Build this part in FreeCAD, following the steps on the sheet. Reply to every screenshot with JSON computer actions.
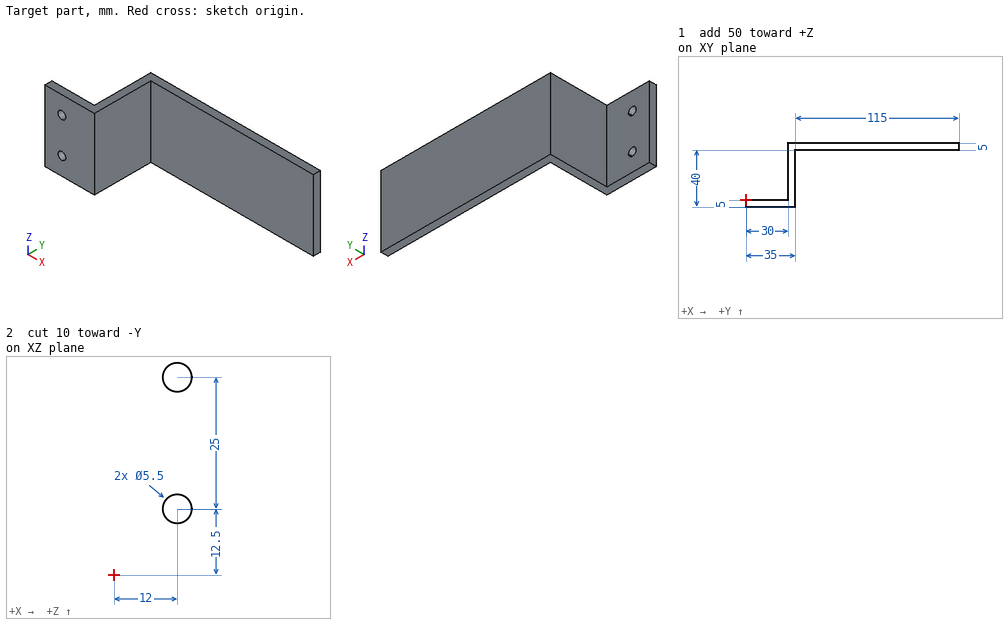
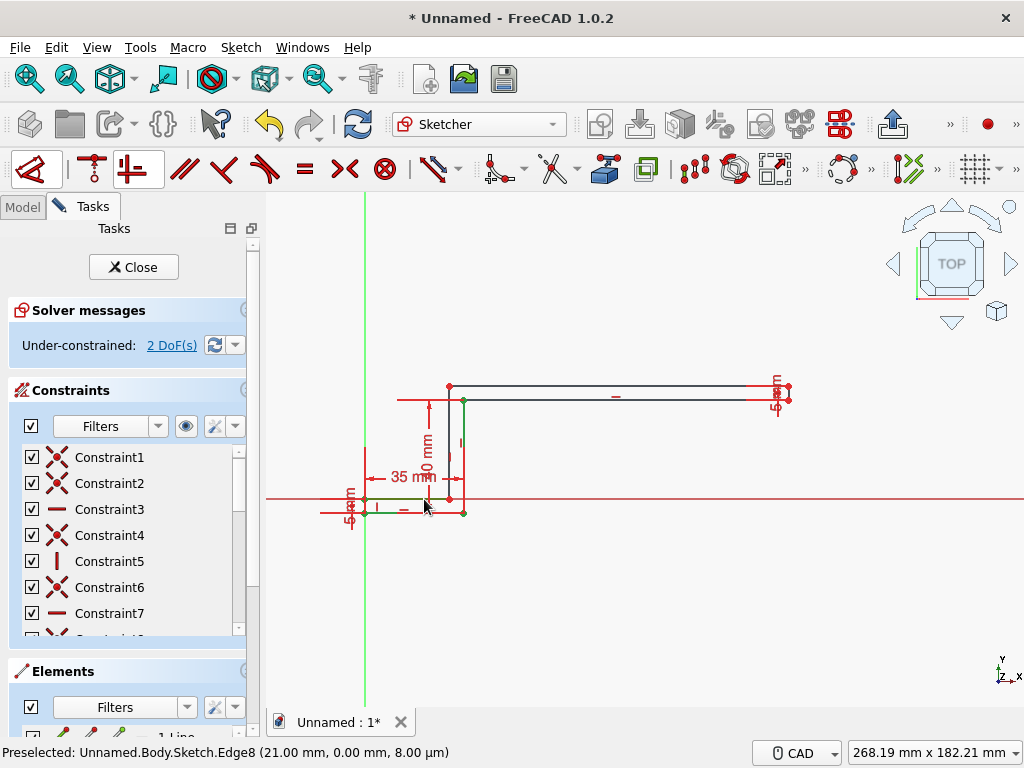
{"action": "key", "text": "l"}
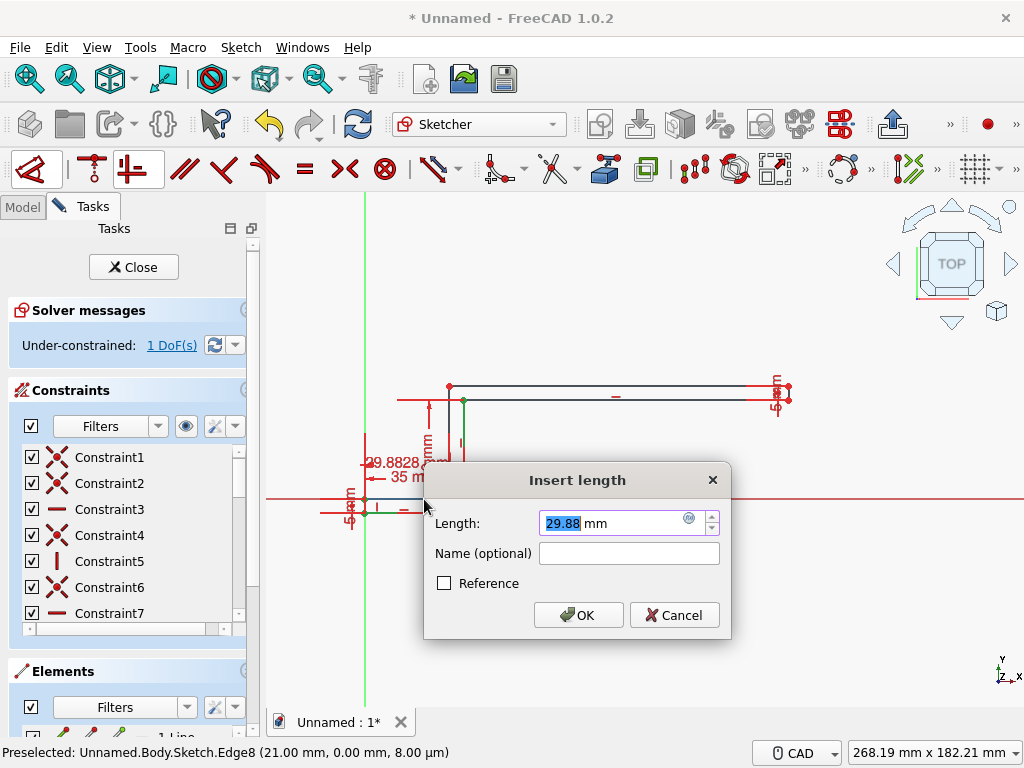
{"action": "type", "text": "30"}
{"action": "key", "text": "Return"}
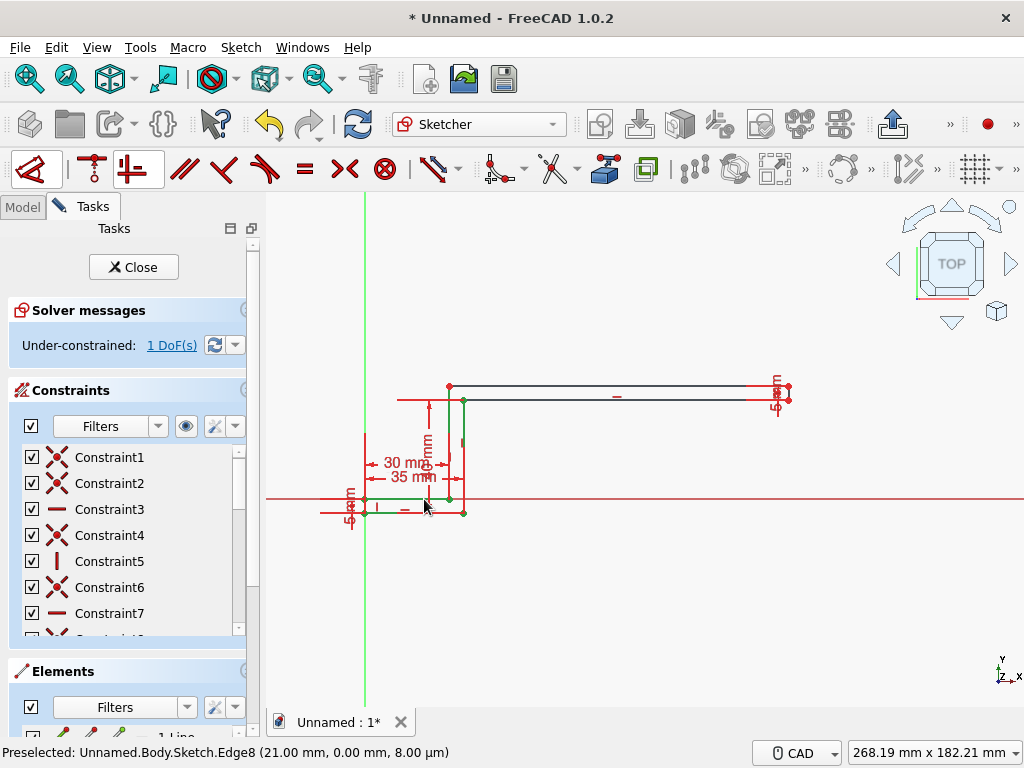
{"action": "left_click", "coordinate": [561, 400]}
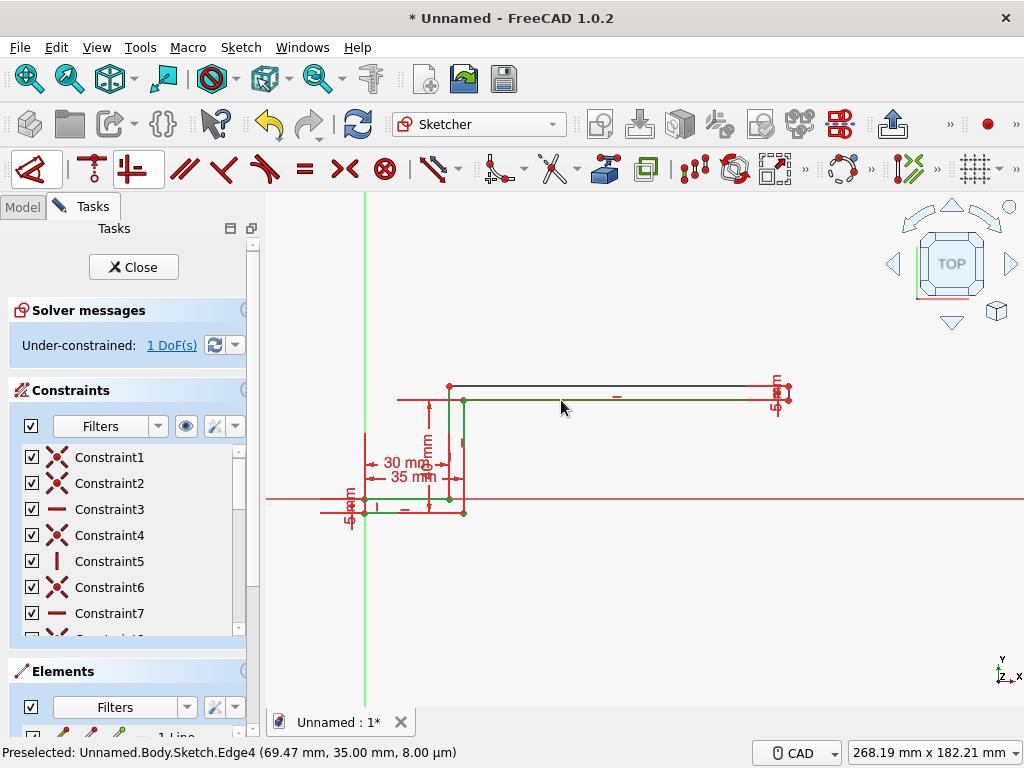
{"action": "left_click", "coordinate": [56, 170]}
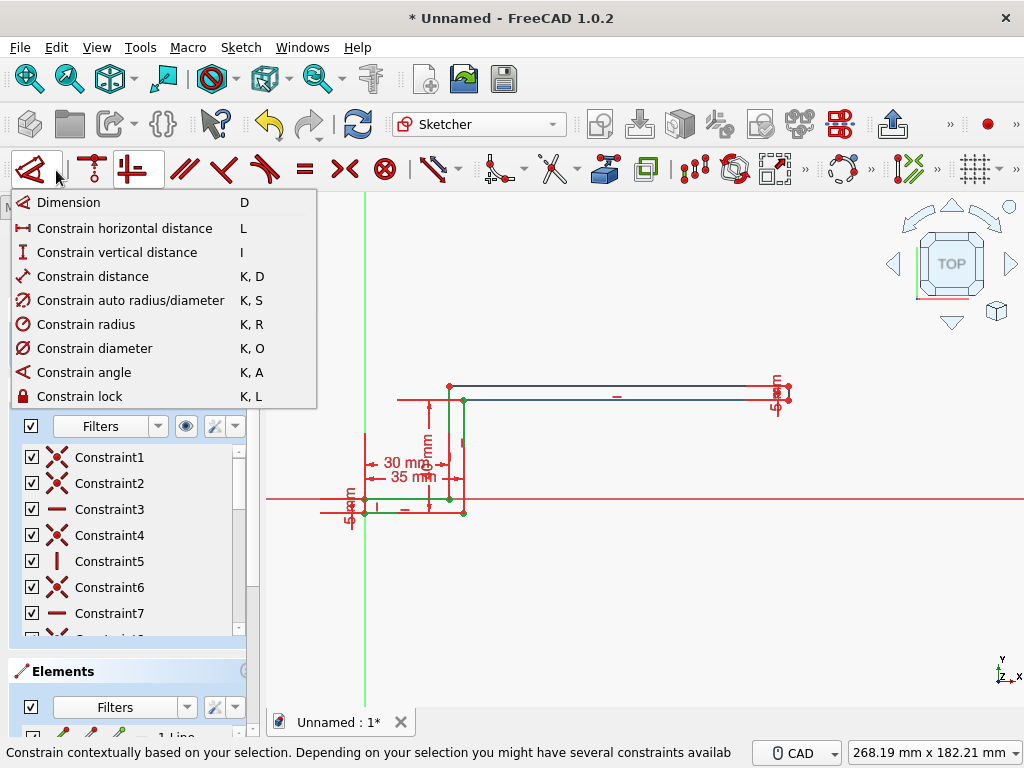
{"action": "left_click", "coordinate": [164, 228]}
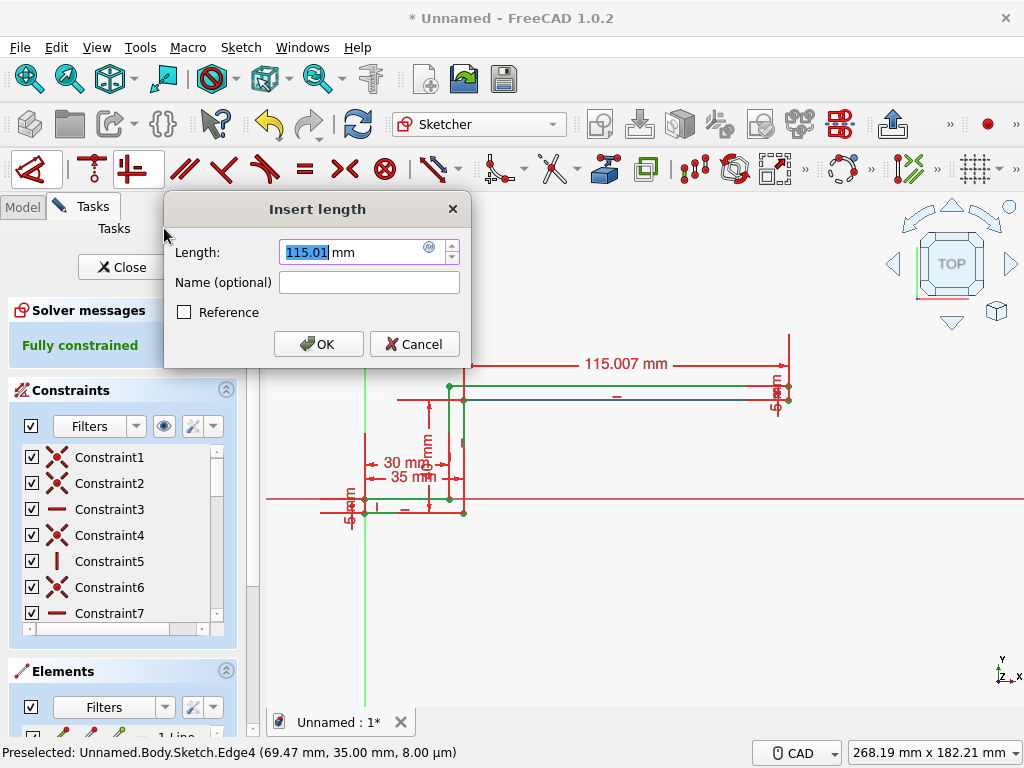
{"action": "type", "text": "115"}
{"action": "key", "text": "Return"}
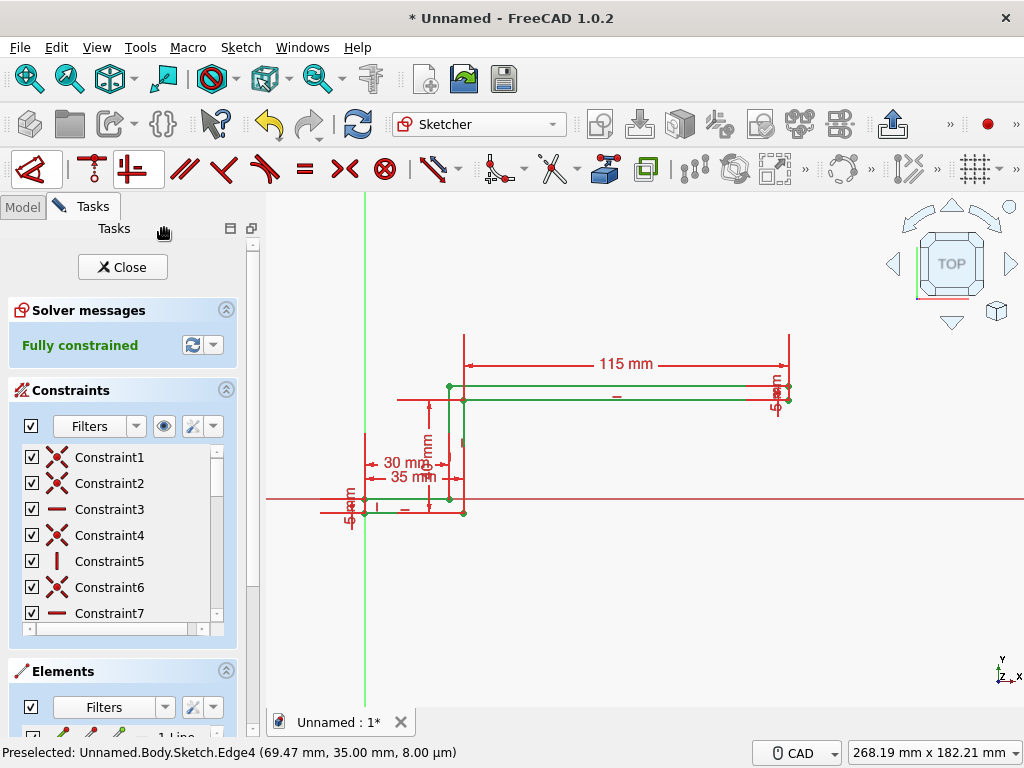
{"action": "left_click", "coordinate": [123, 267]}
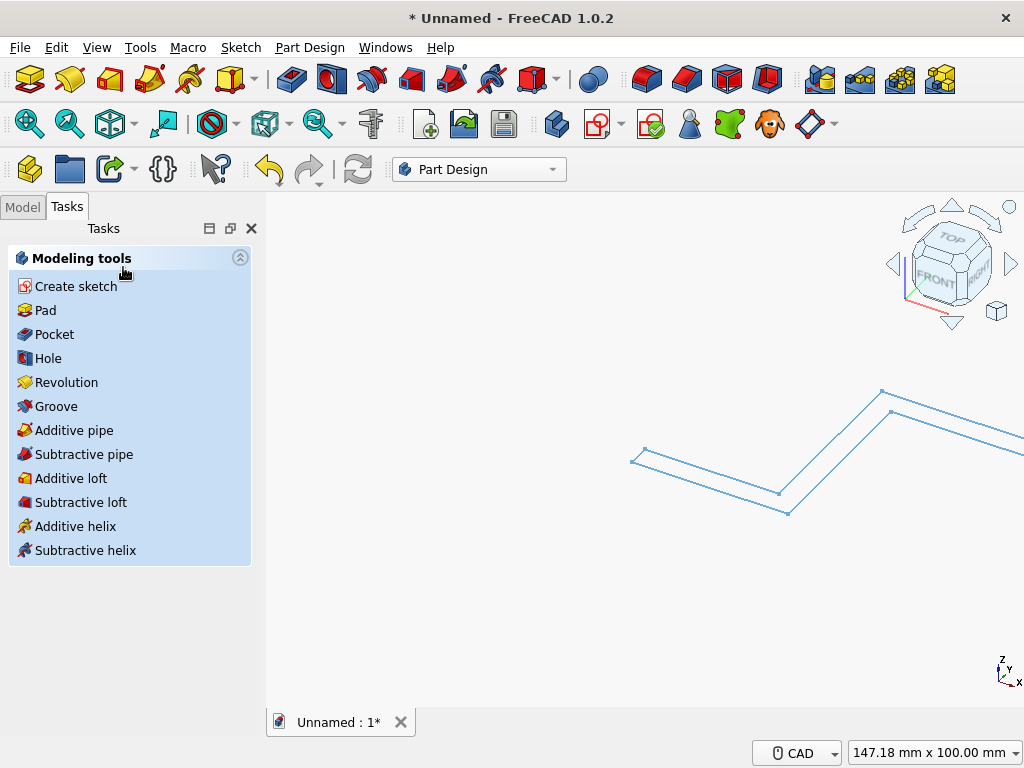
{"action": "left_click", "coordinate": [30, 80]}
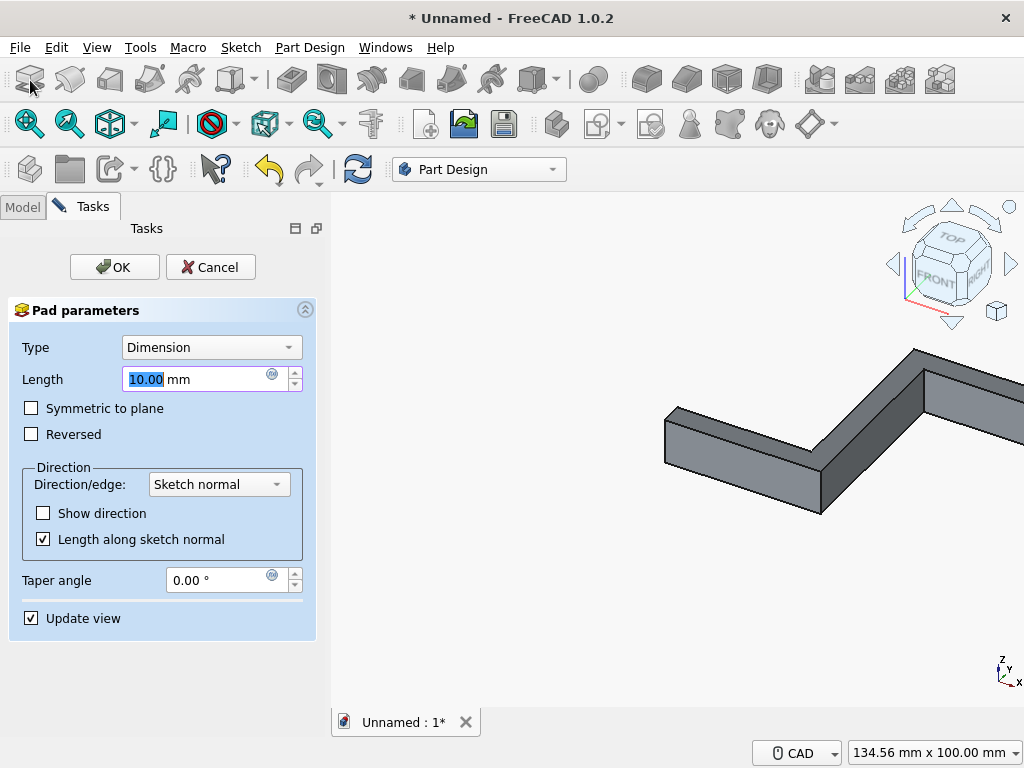
{"action": "type", "text": "50"}
{"action": "key", "text": "Tab"}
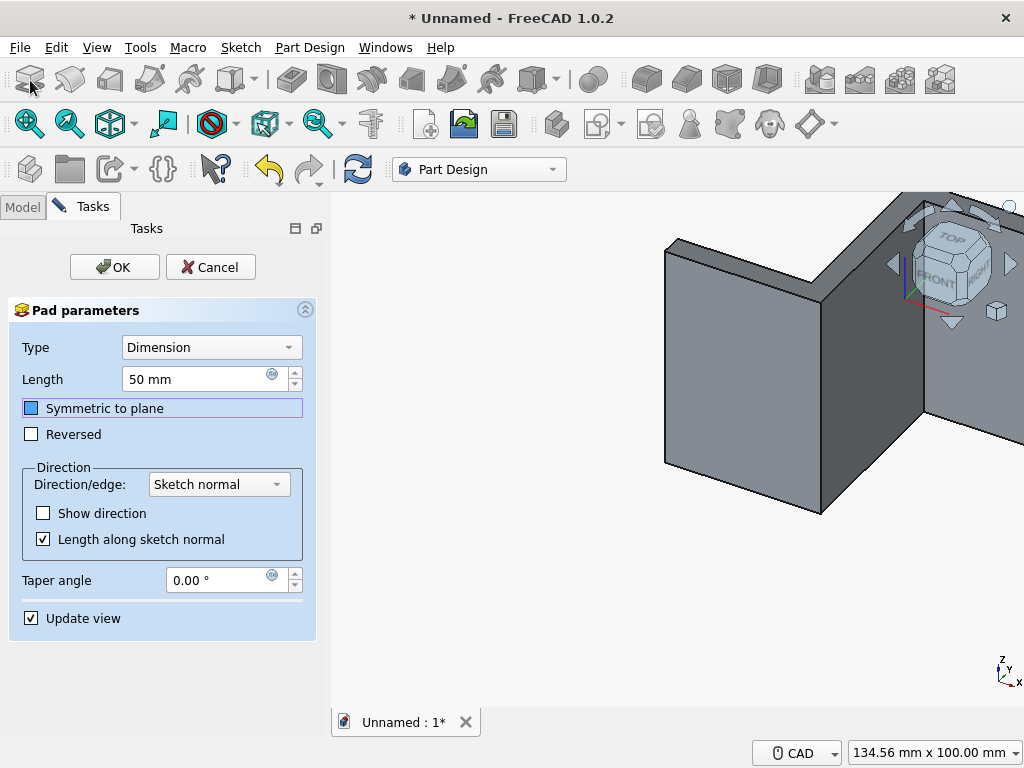
{"action": "left_click", "coordinate": [115, 267]}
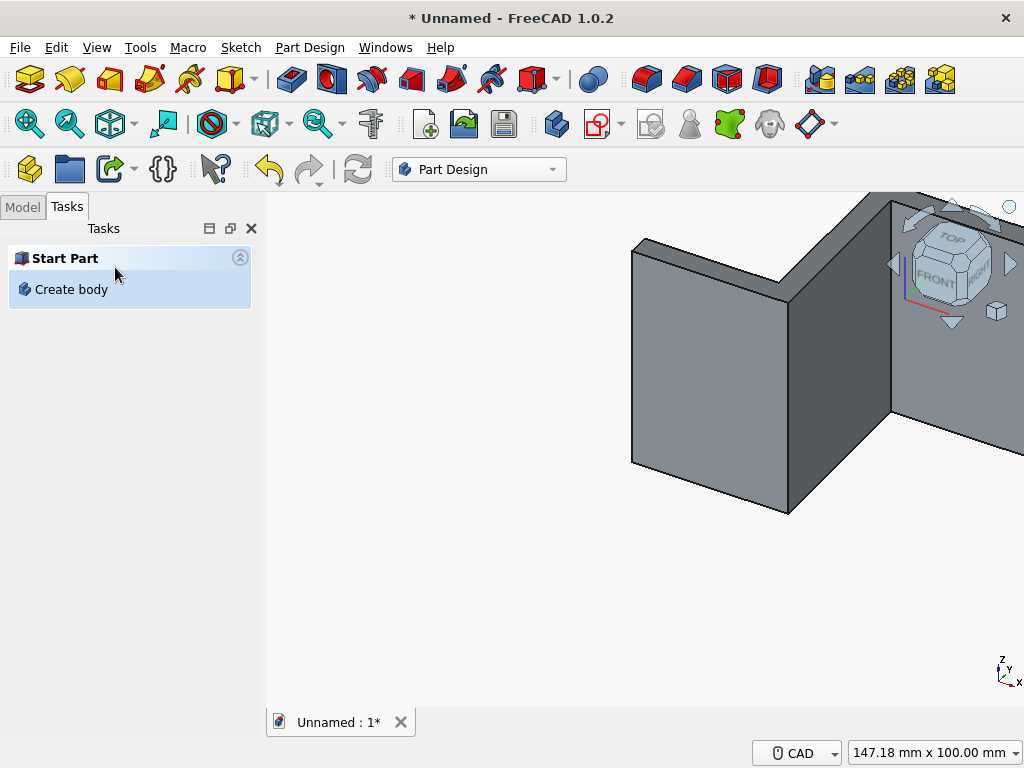
{"action": "left_click", "coordinate": [30, 124]}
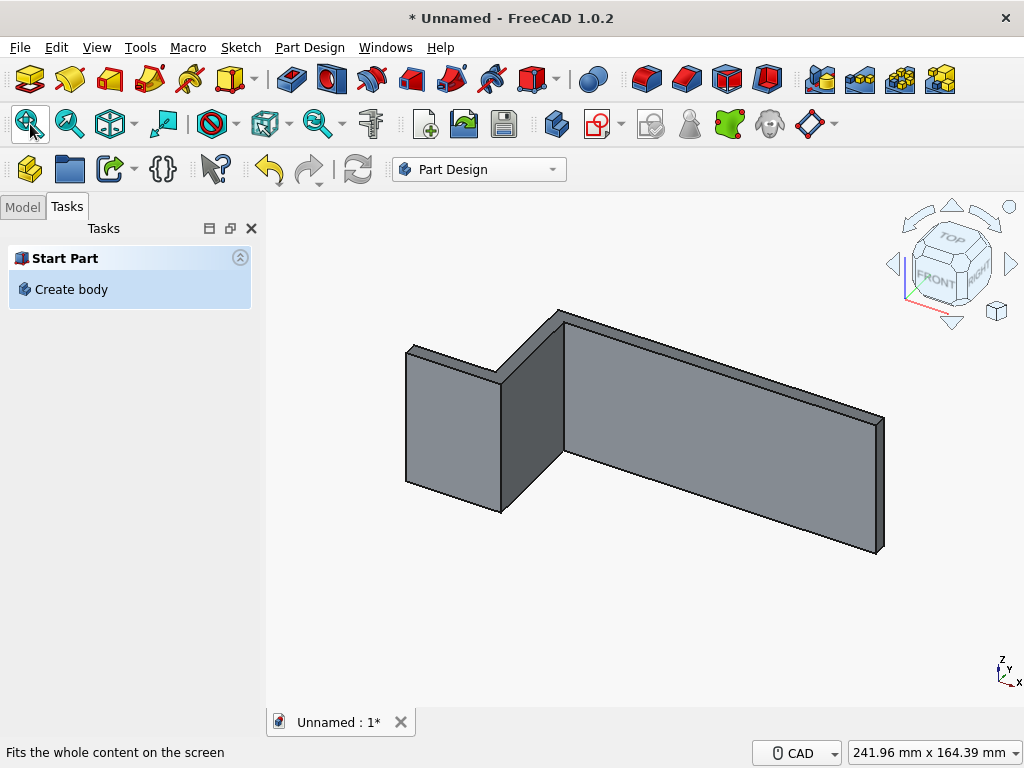
{"action": "left_click", "coordinate": [598, 124]}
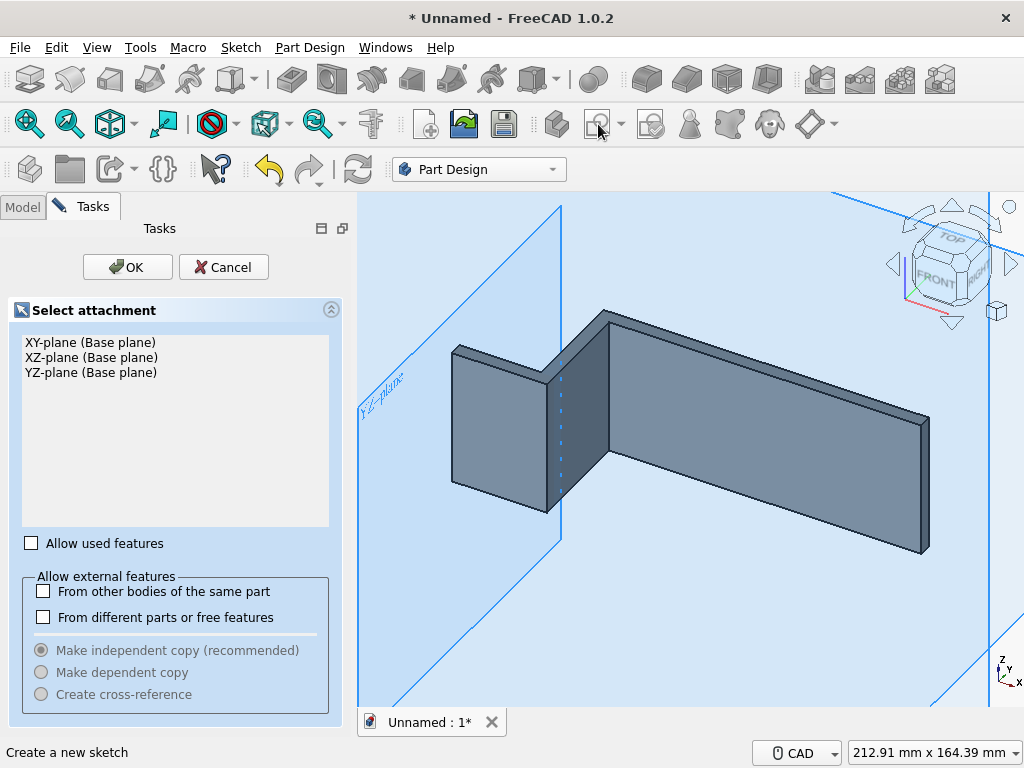
{"action": "left_click", "coordinate": [82, 358]}